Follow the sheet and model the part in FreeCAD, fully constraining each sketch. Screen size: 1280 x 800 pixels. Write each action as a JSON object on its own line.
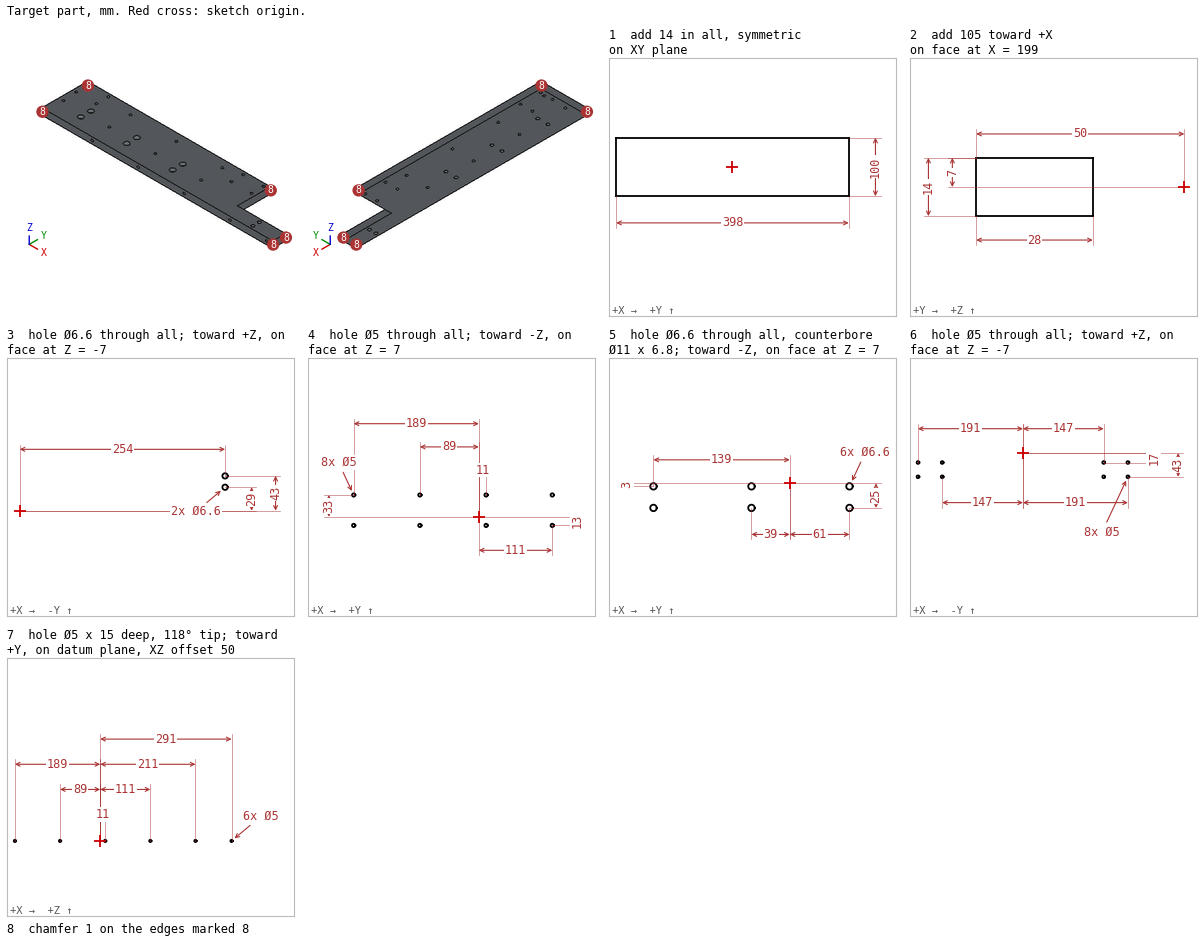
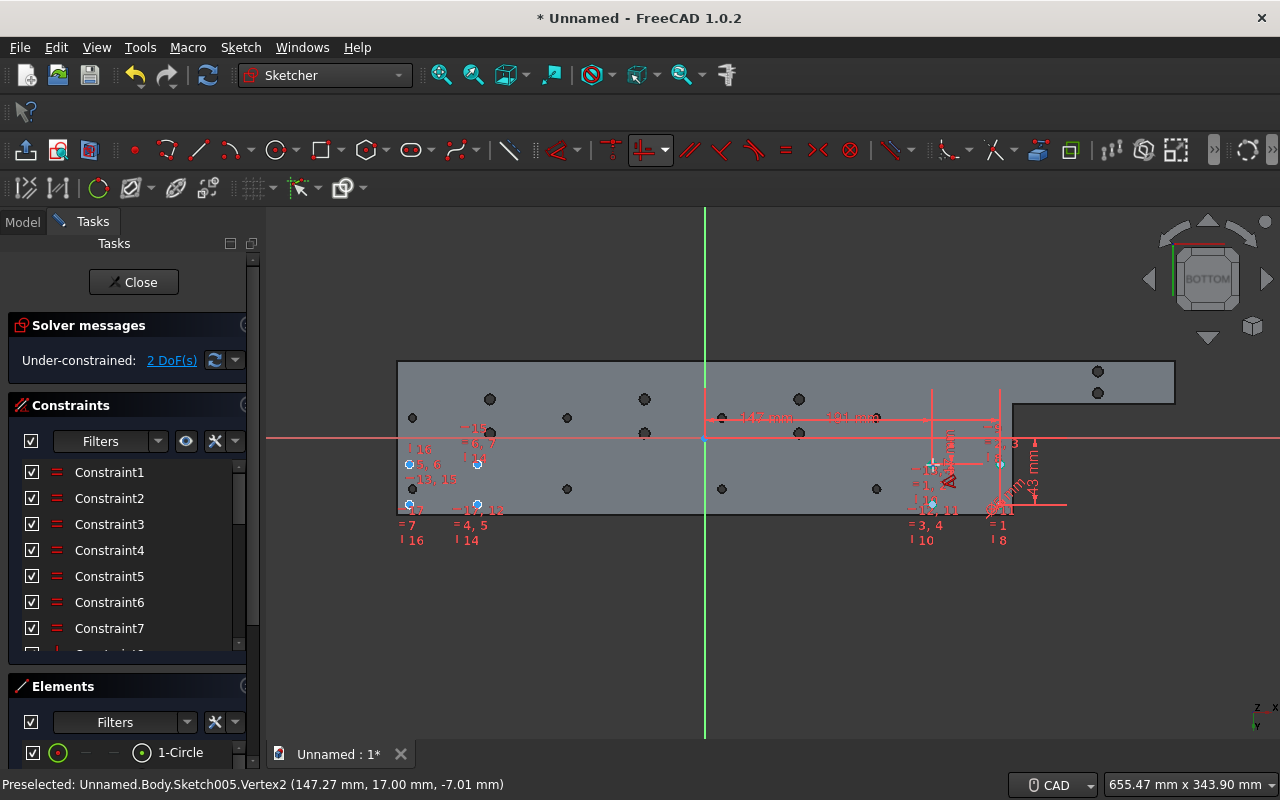
{"action": "left_click", "coordinate": [478, 505]}
{"action": "left_click", "coordinate": [591, 404]}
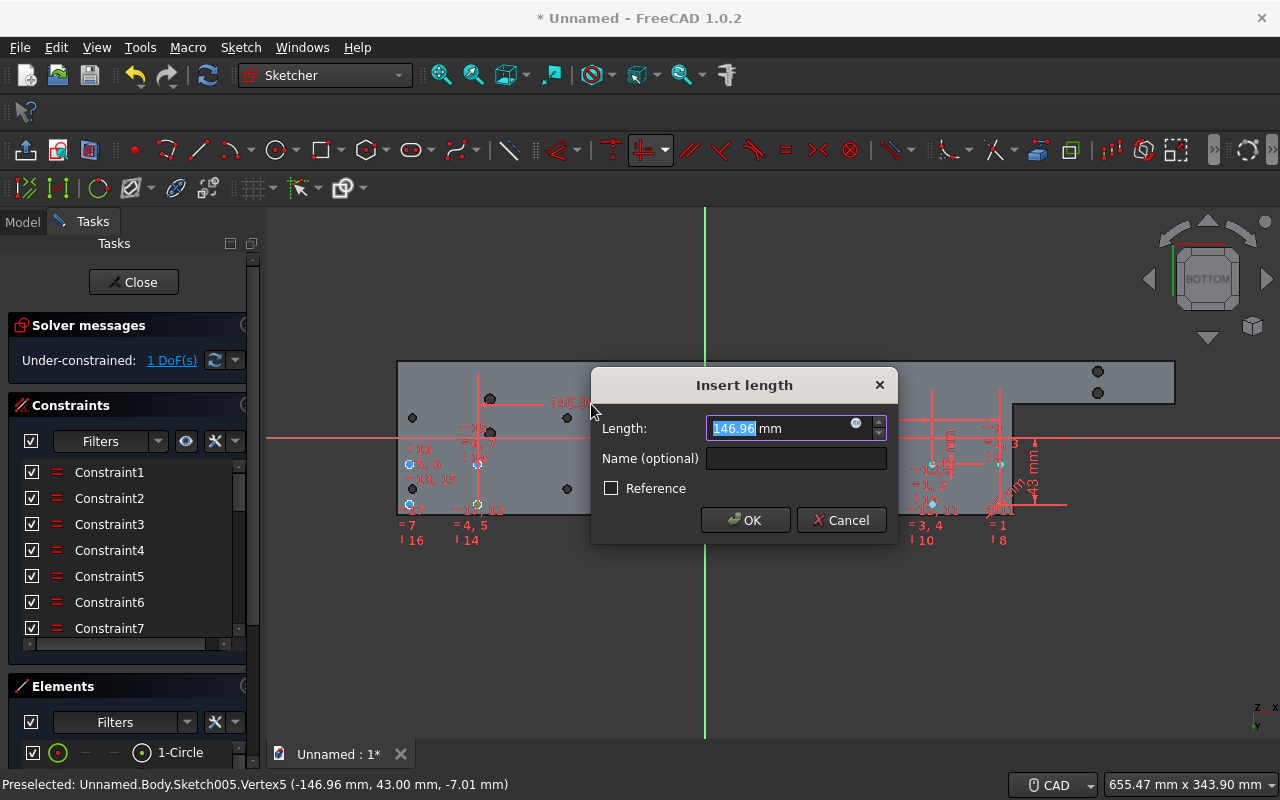
{"action": "type", "text": "147"}
{"action": "key", "text": "Return"}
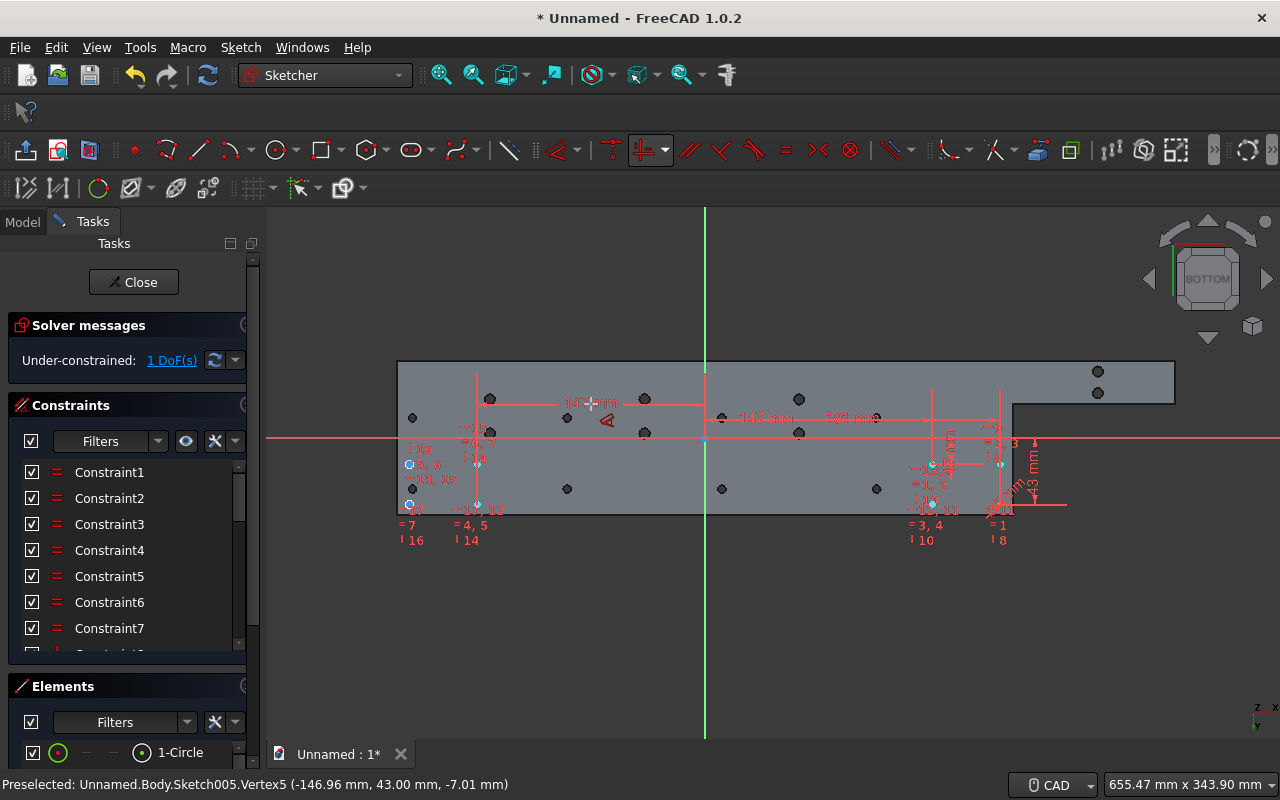
{"action": "left_click", "coordinate": [410, 464]}
{"action": "left_click", "coordinate": [489, 404]}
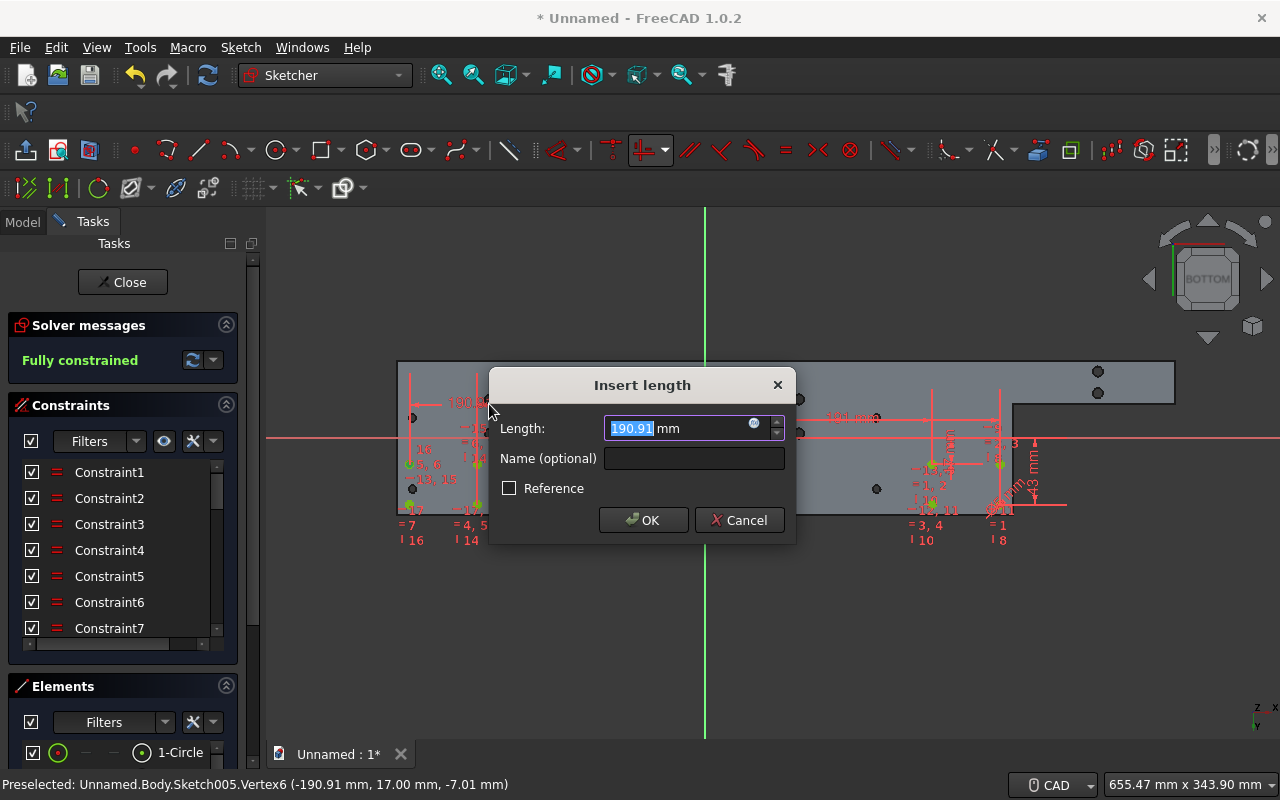
{"action": "type", "text": "191"}
{"action": "key", "text": "Return"}
{"action": "key", "text": "Escape"}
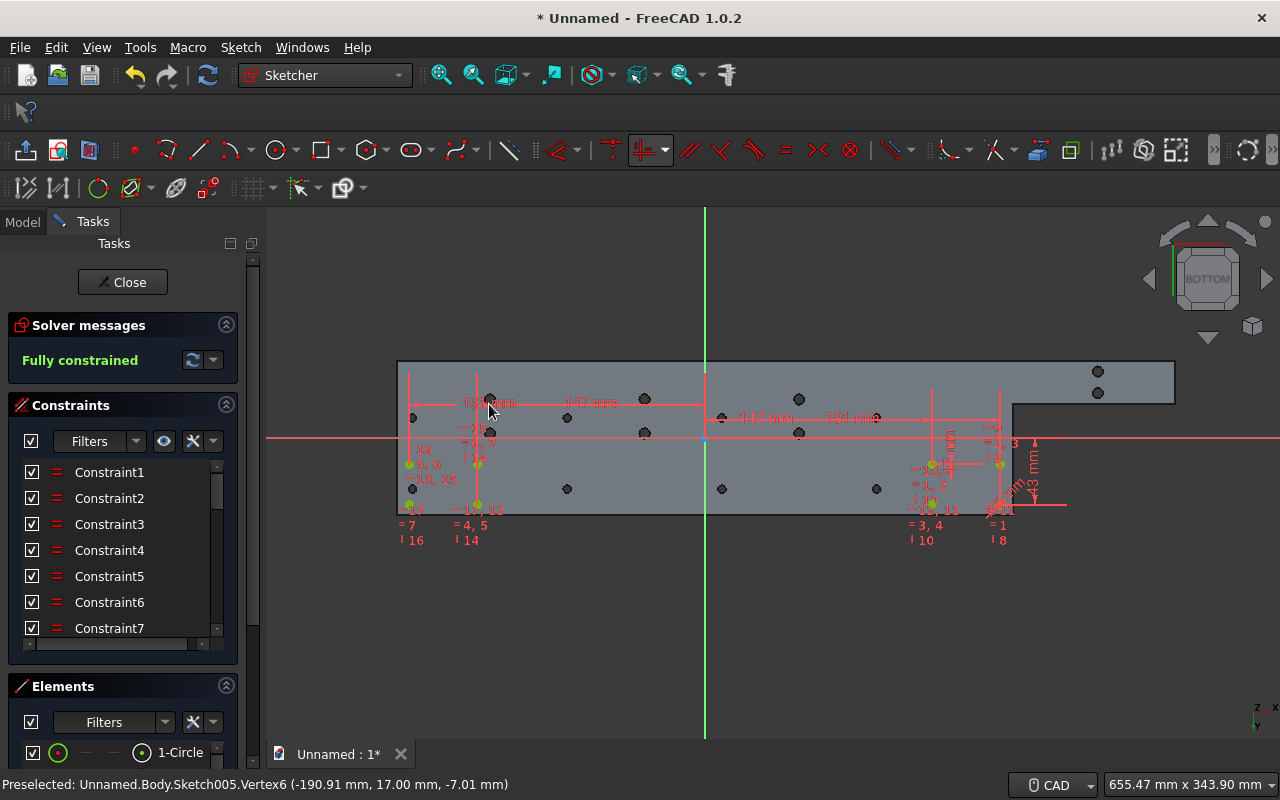
{"action": "left_click", "coordinate": [123, 282]}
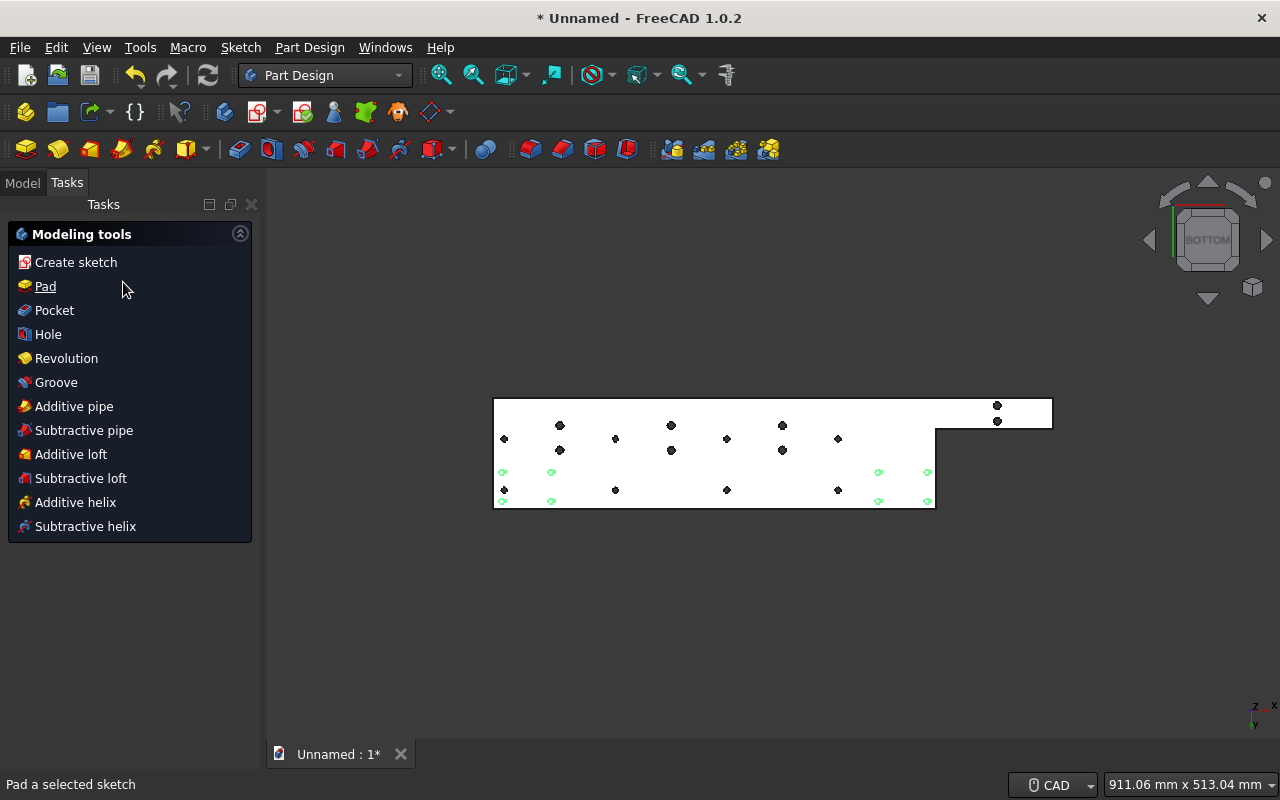
{"action": "left_click", "coordinate": [272, 150]}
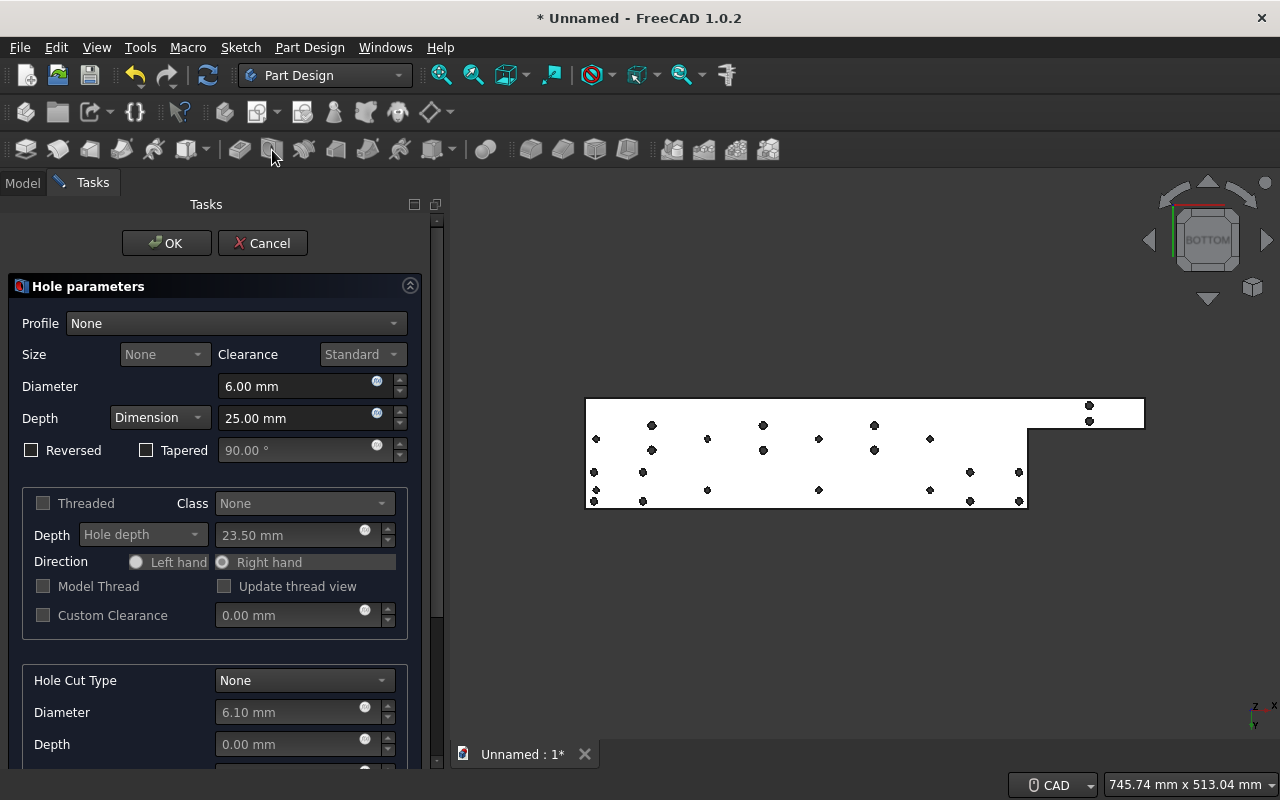
{"action": "triple_click", "coordinate": [305, 386]}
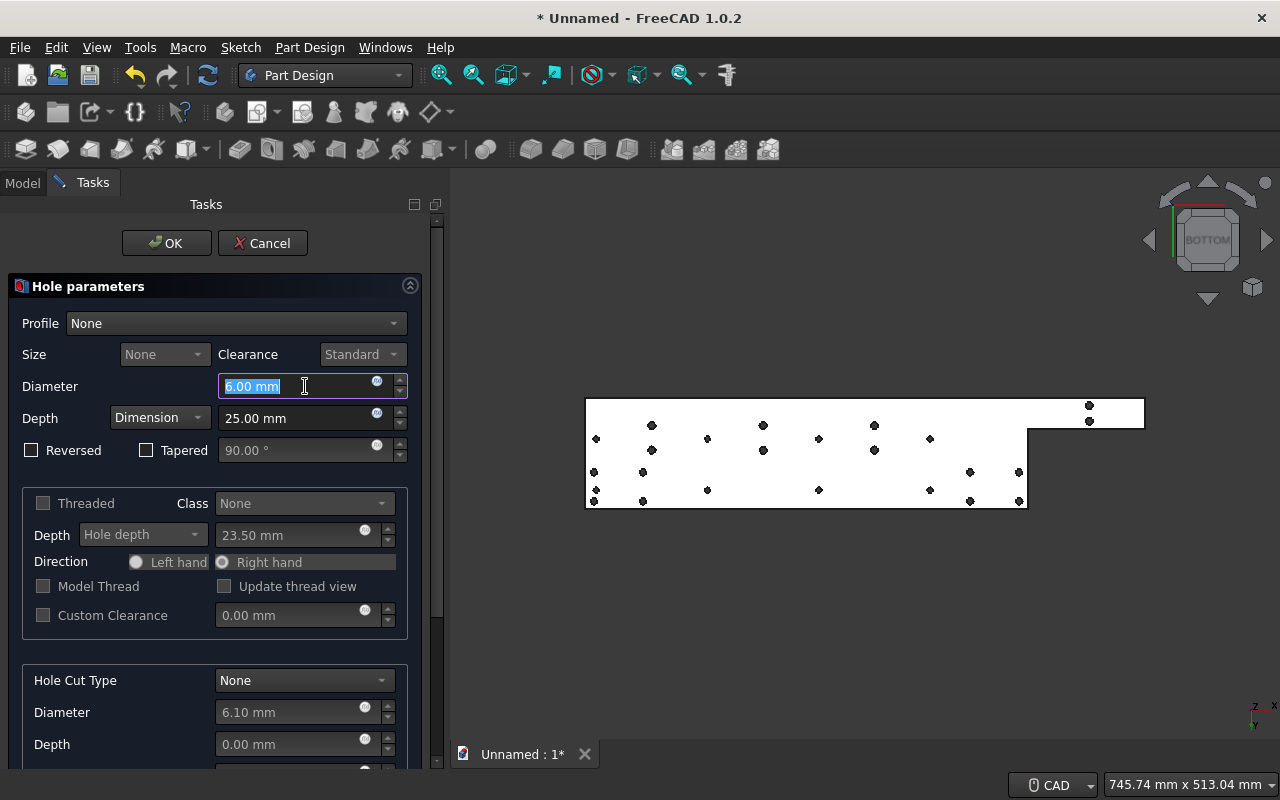
{"action": "type", "text": "5"}
{"action": "key", "text": "Tab"}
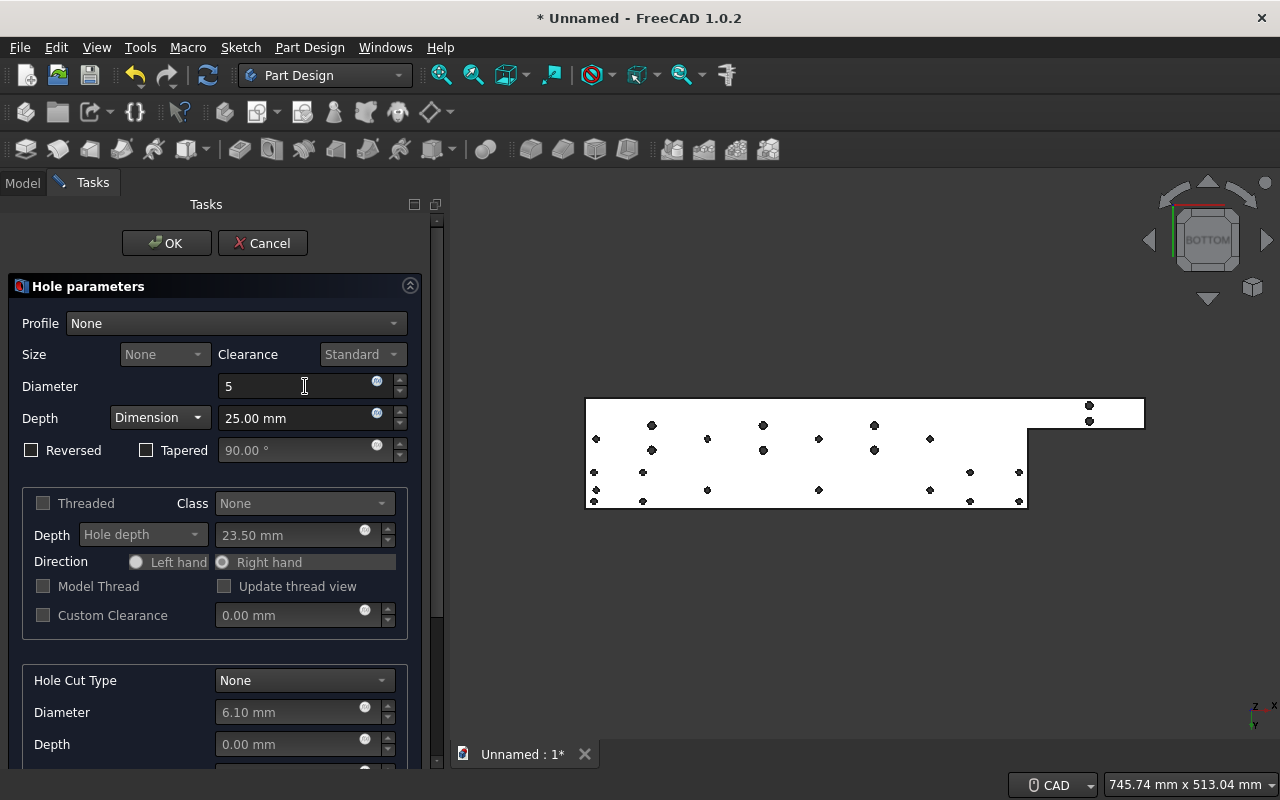
{"action": "left_click", "coordinate": [161, 418]}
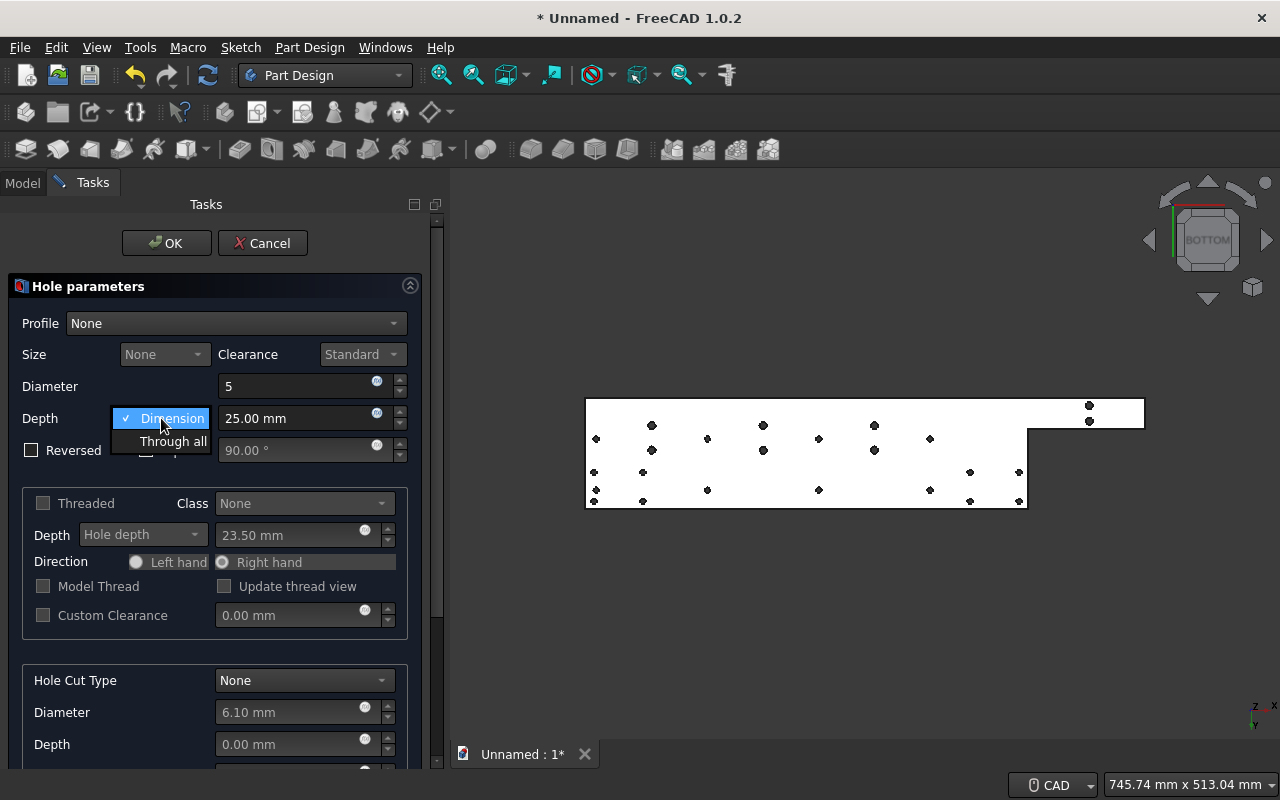
{"action": "left_click", "coordinate": [160, 442]}